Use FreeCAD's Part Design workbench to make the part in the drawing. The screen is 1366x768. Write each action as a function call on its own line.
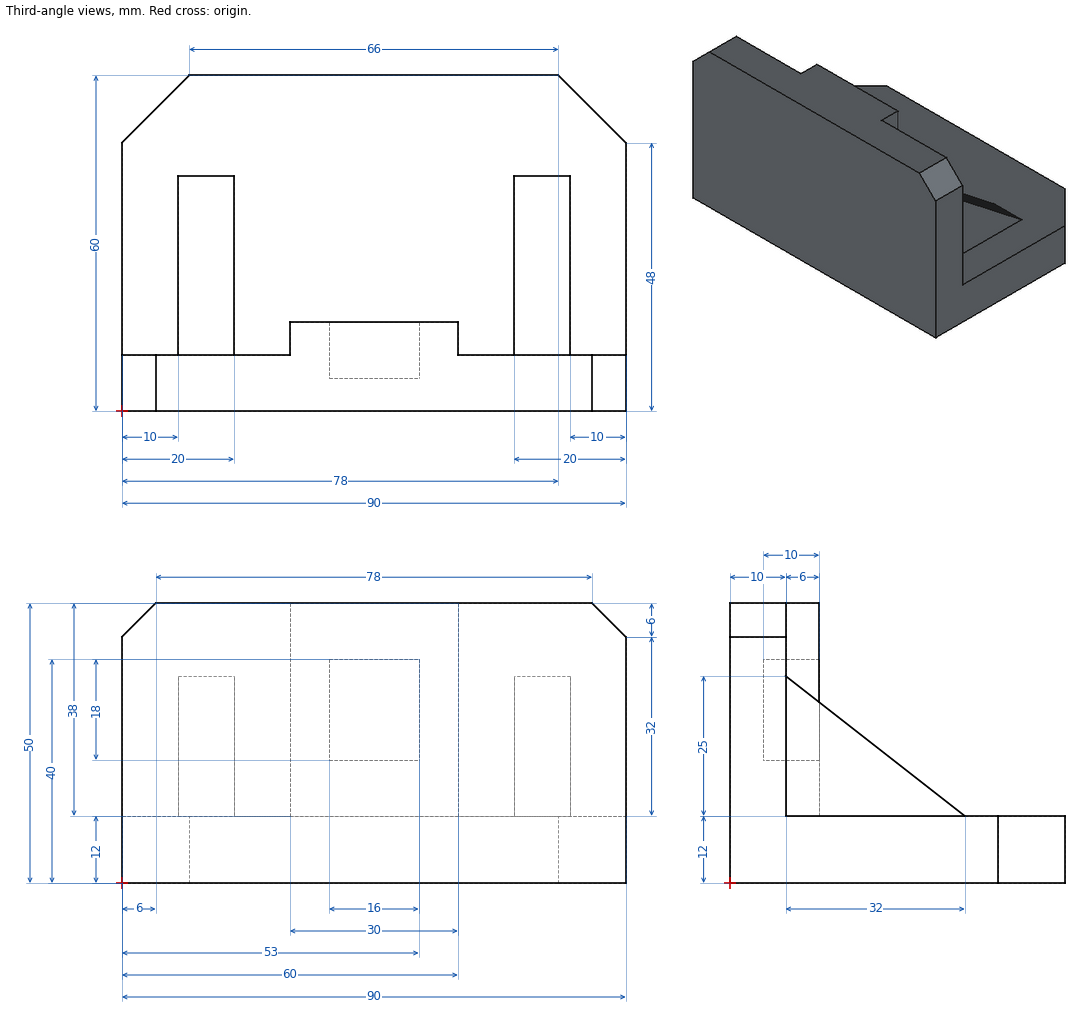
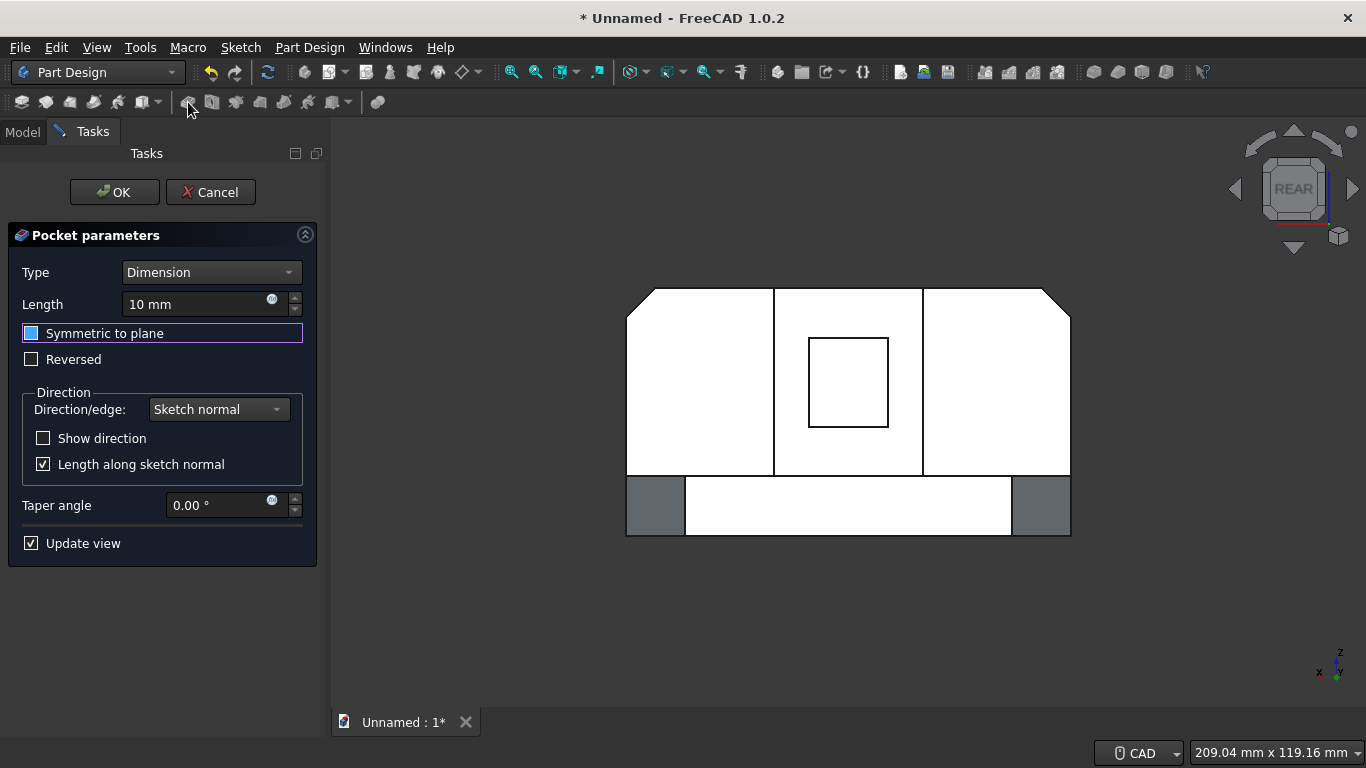
click(115, 192)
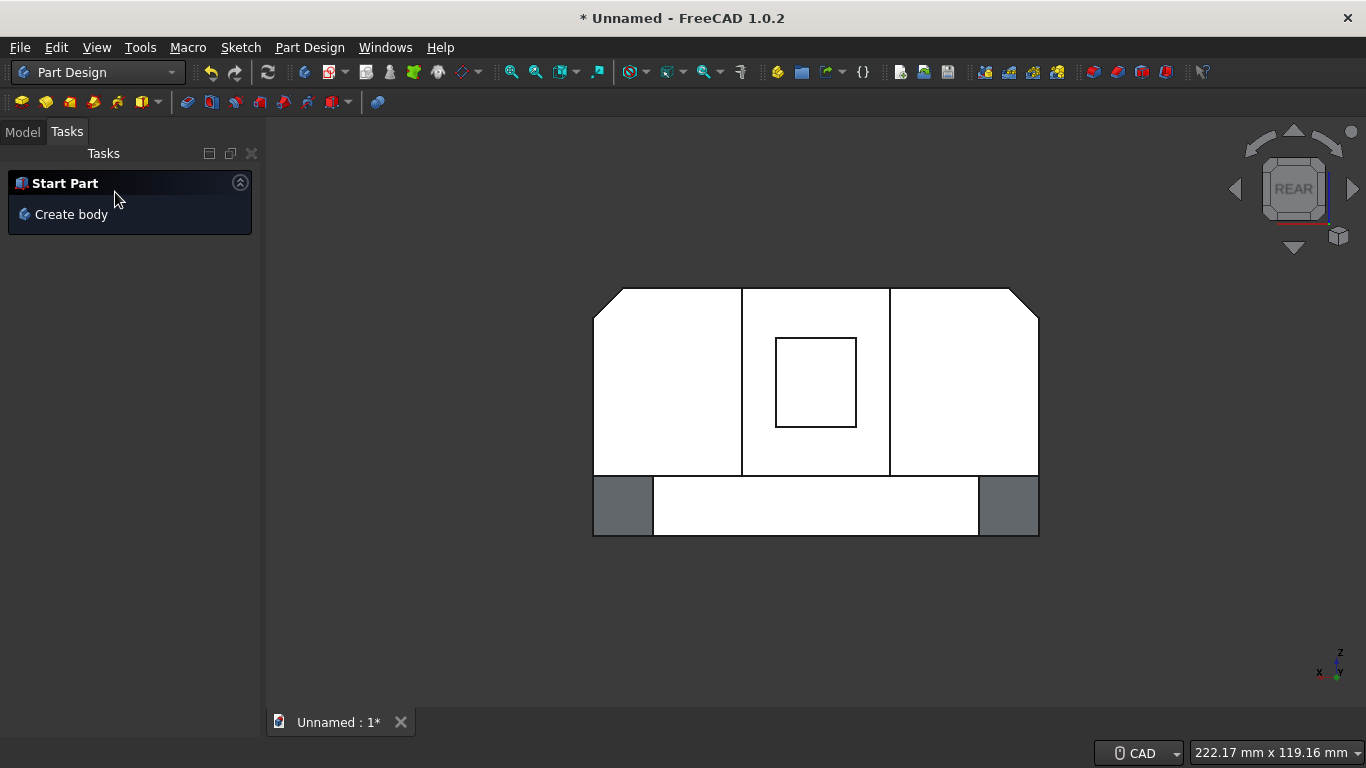
click(512, 72)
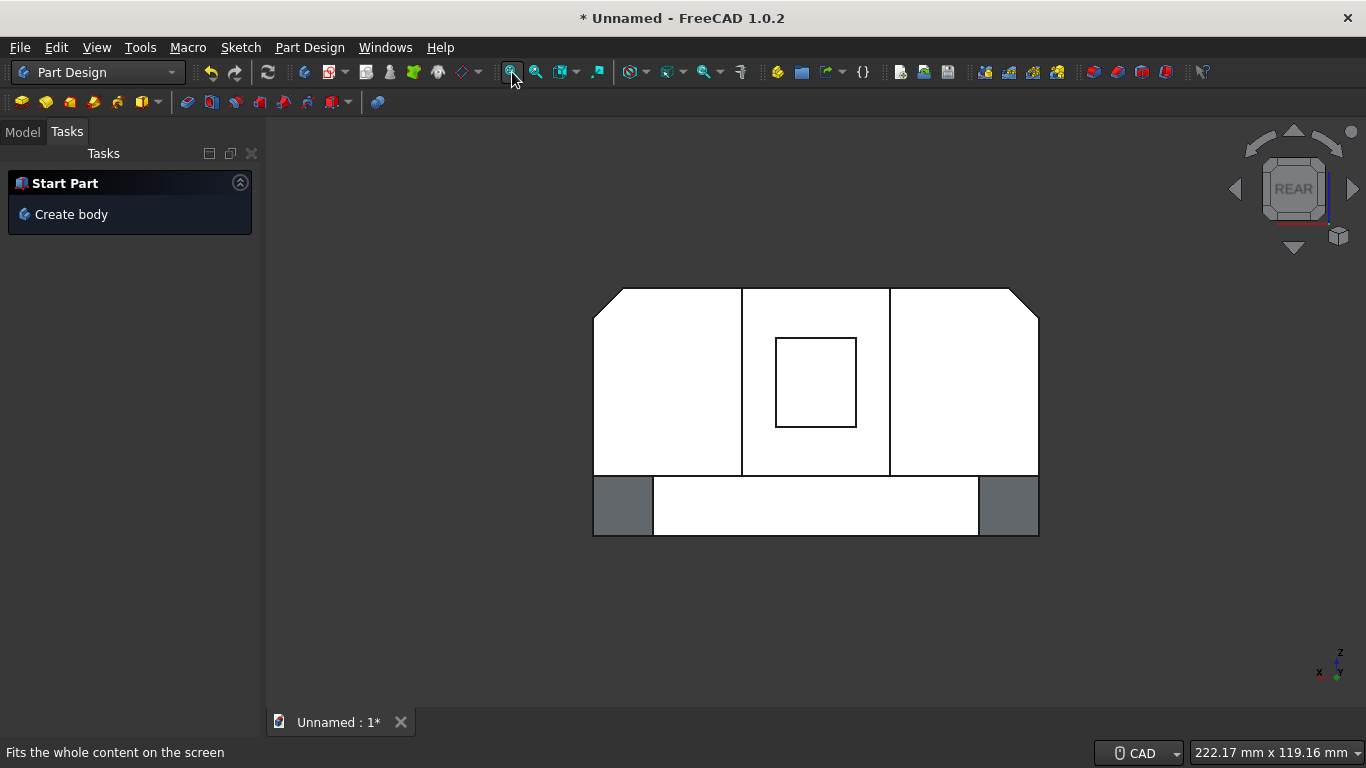
key(6)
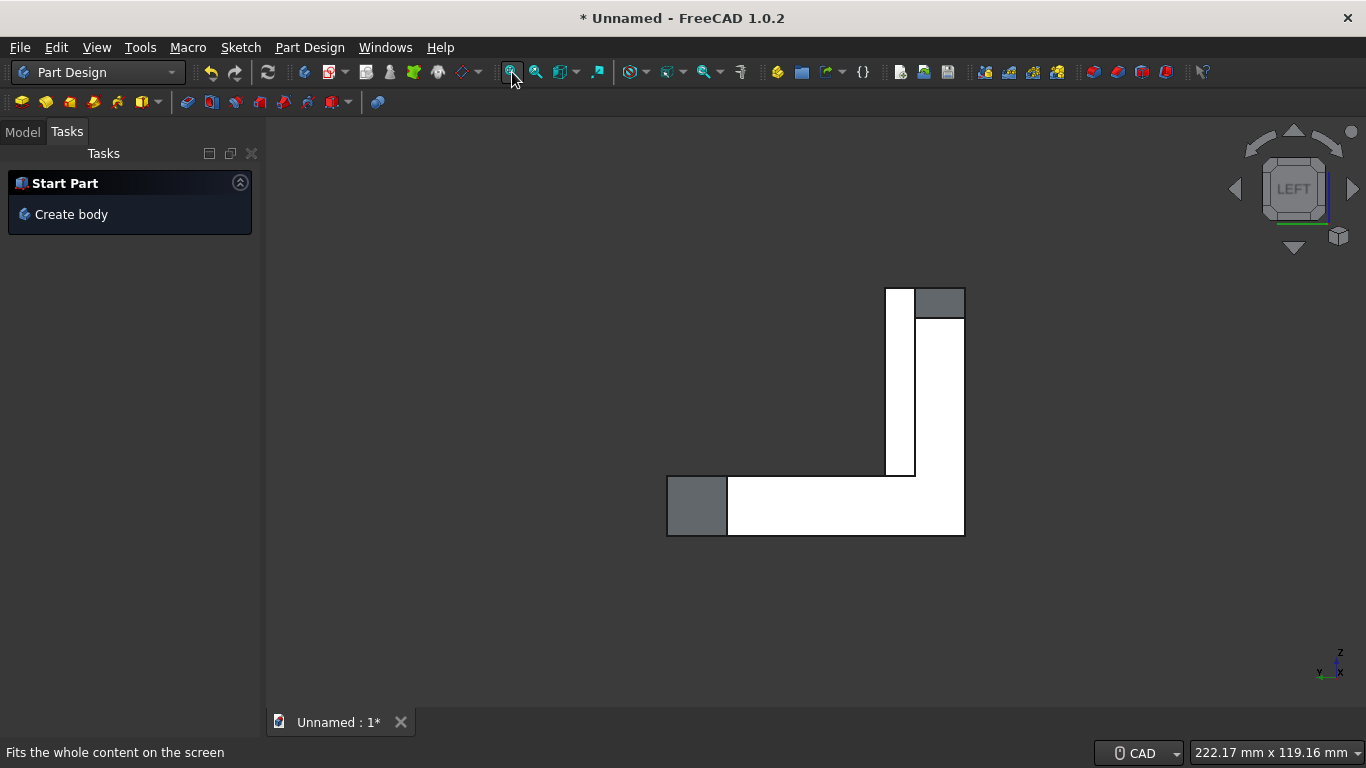
click(512, 72)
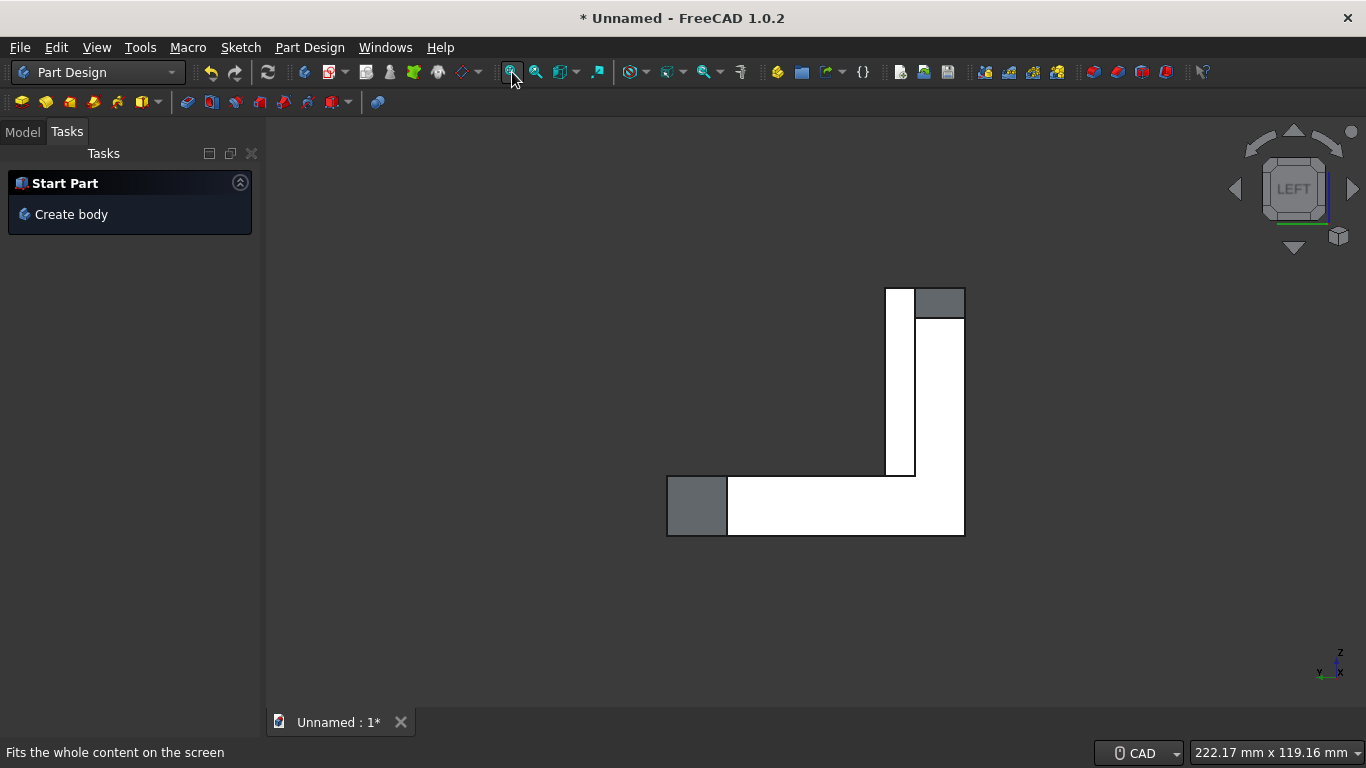
click(948, 488)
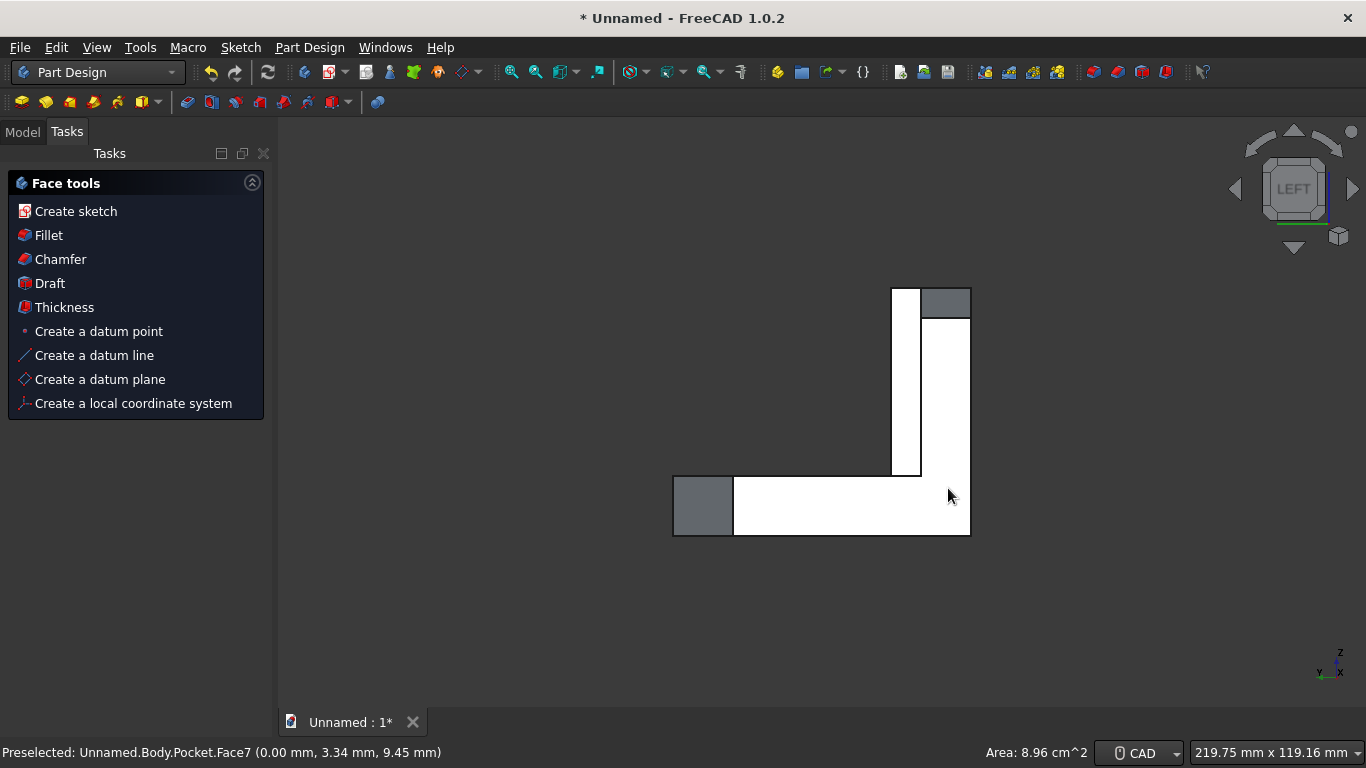
click(330, 72)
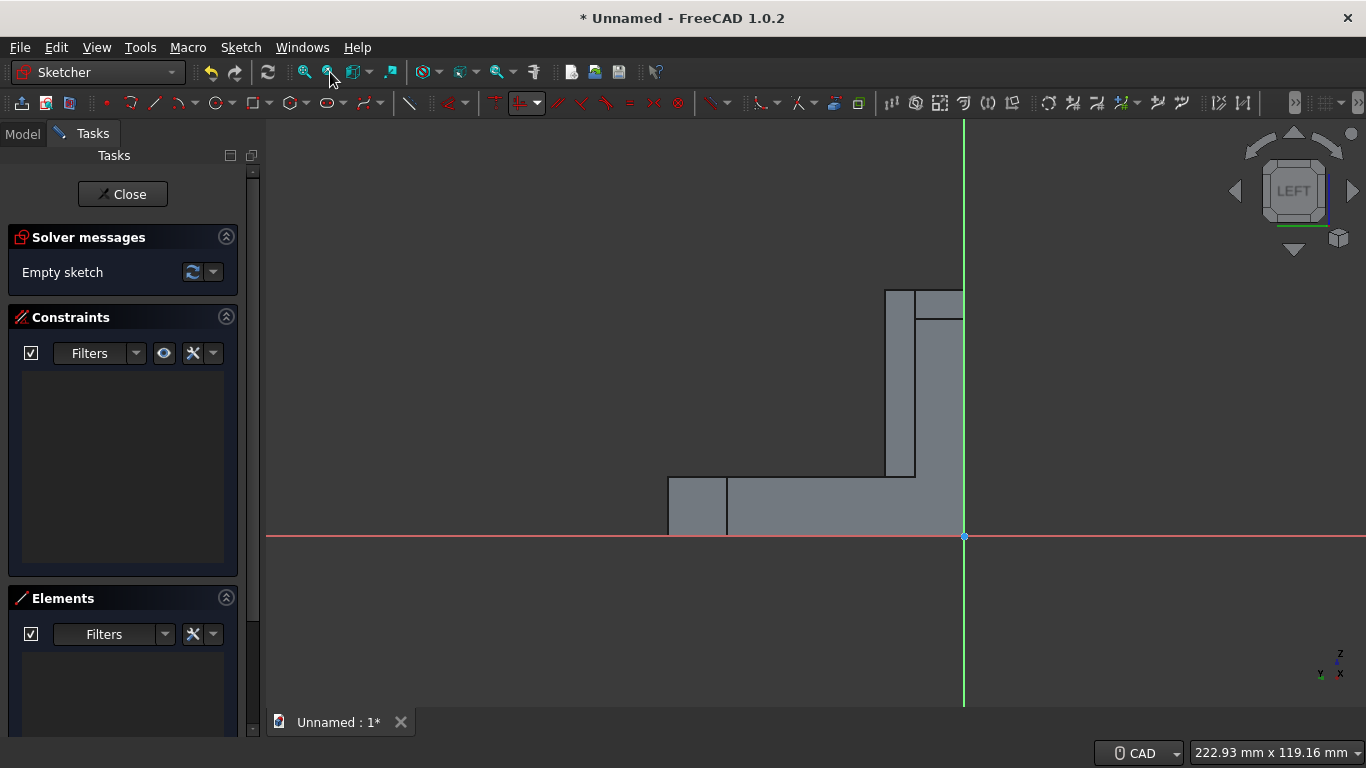
scroll(953, 471, up, 4)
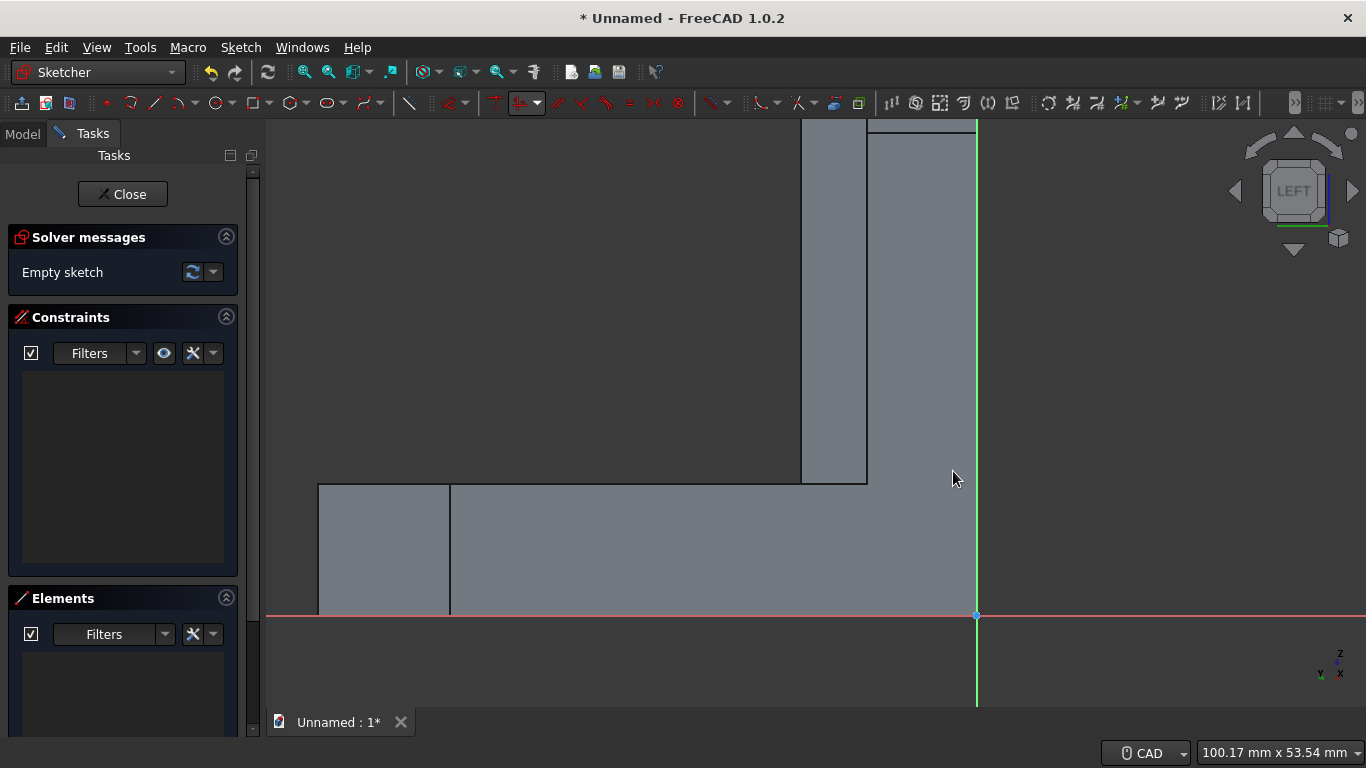
click(132, 104)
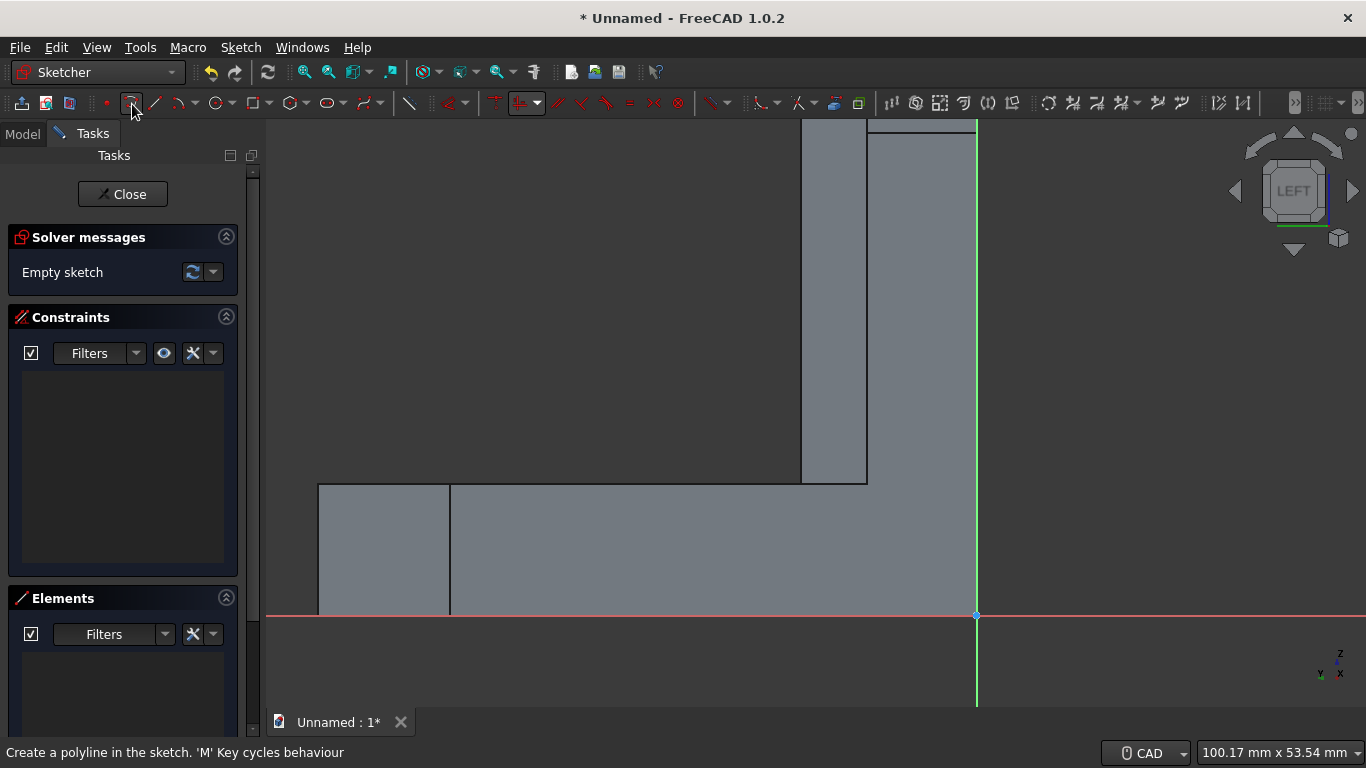
click(867, 484)
click(867, 209)
click(516, 484)
click(867, 485)
key(Escape)
key(Escape)